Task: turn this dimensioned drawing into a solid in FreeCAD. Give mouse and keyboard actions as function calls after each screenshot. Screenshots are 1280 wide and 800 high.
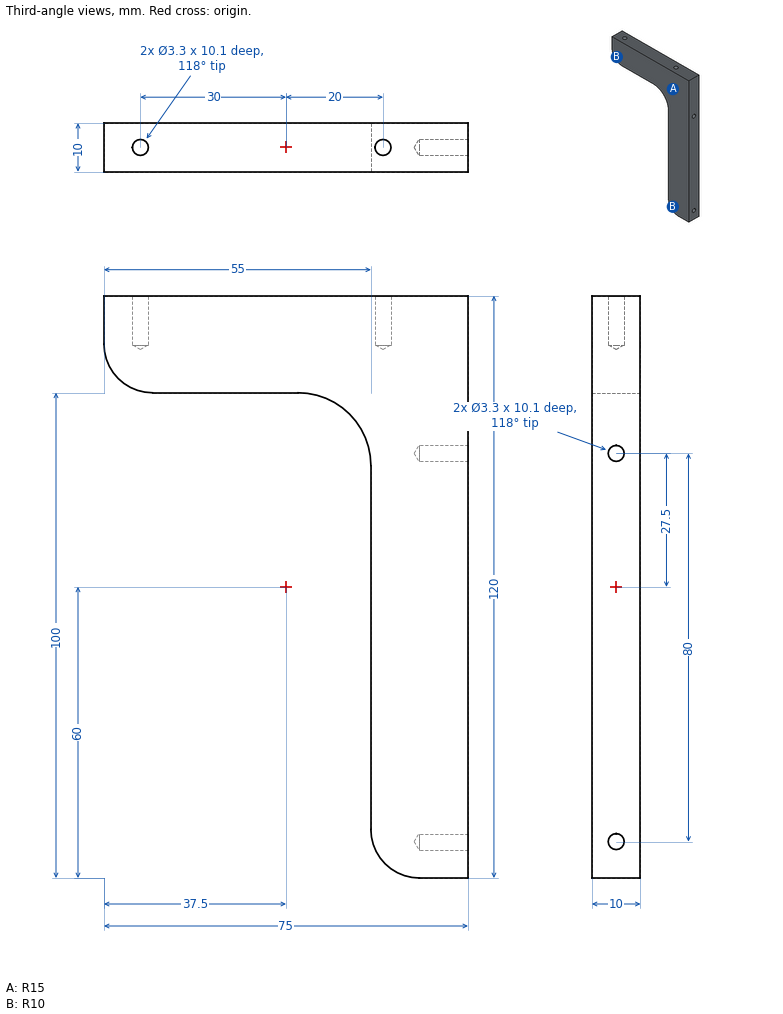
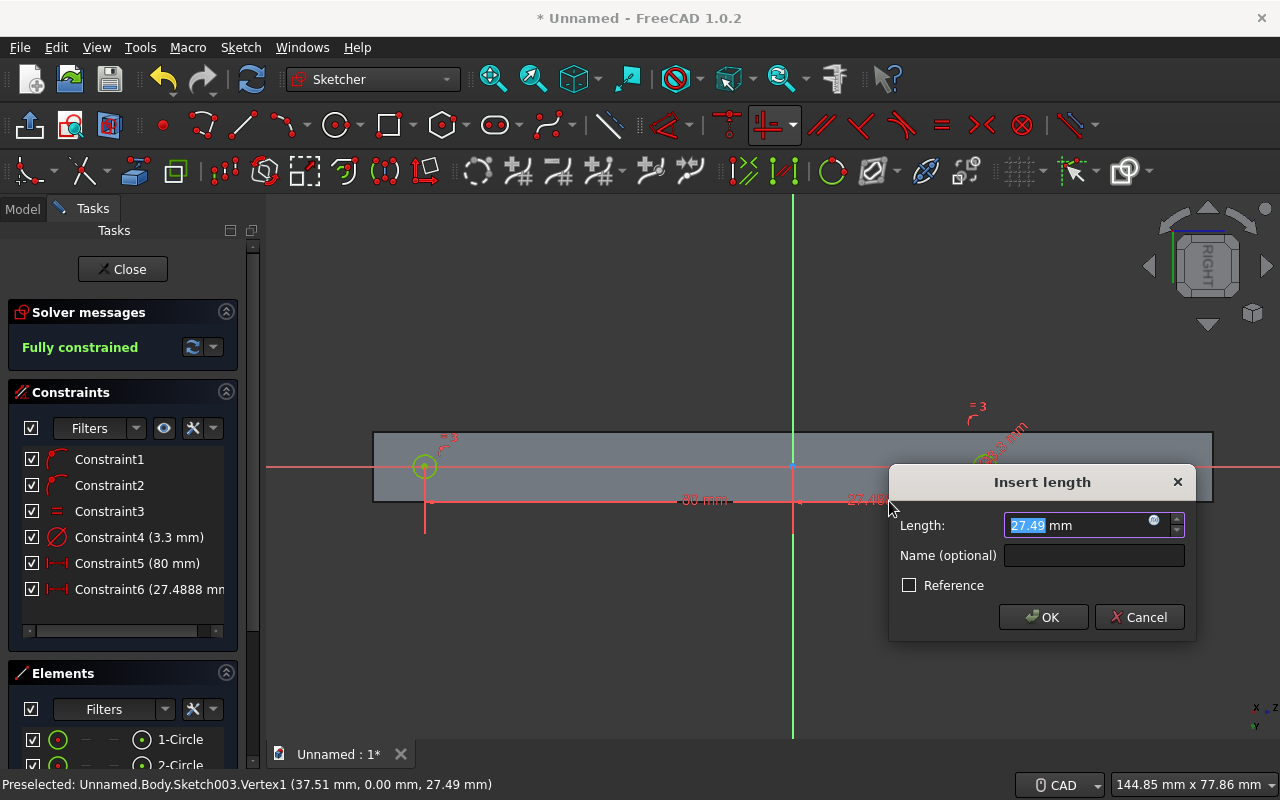
text(27.5)
key(Return)
key(Escape)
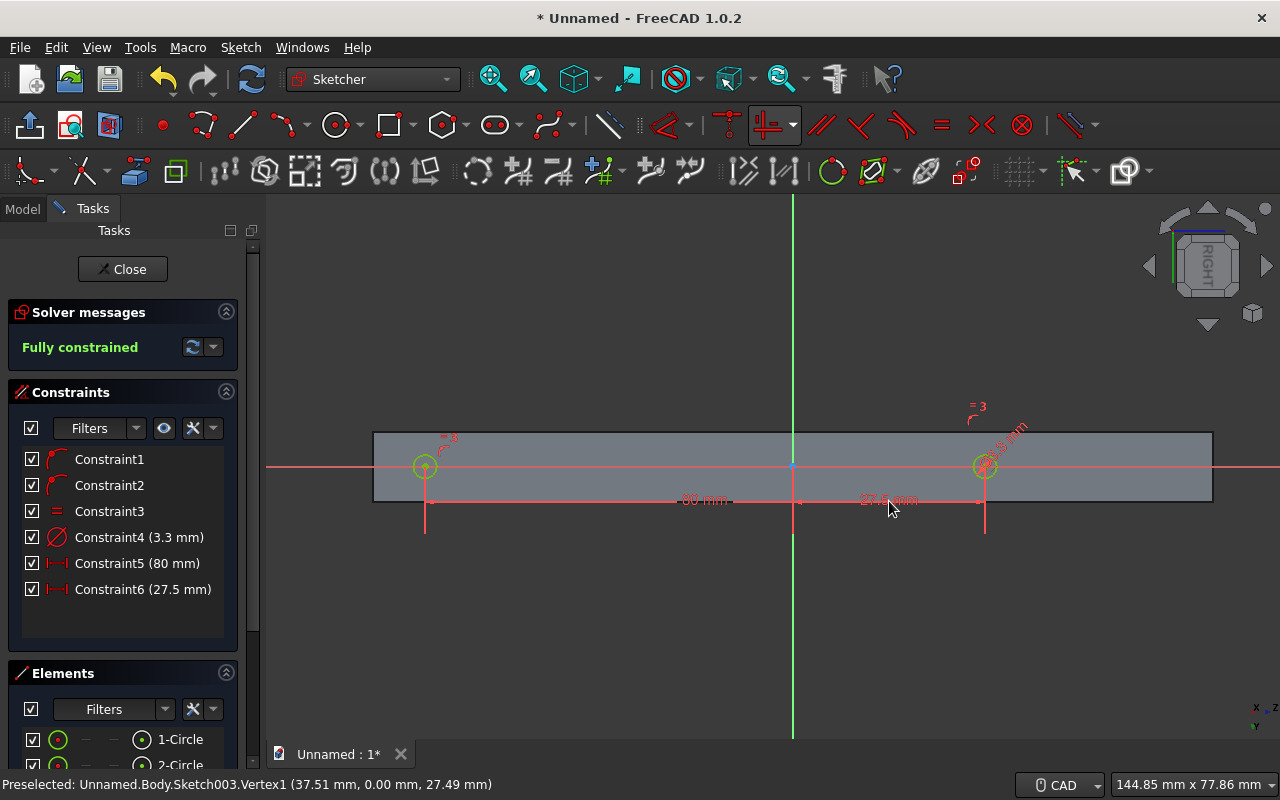
click(123, 269)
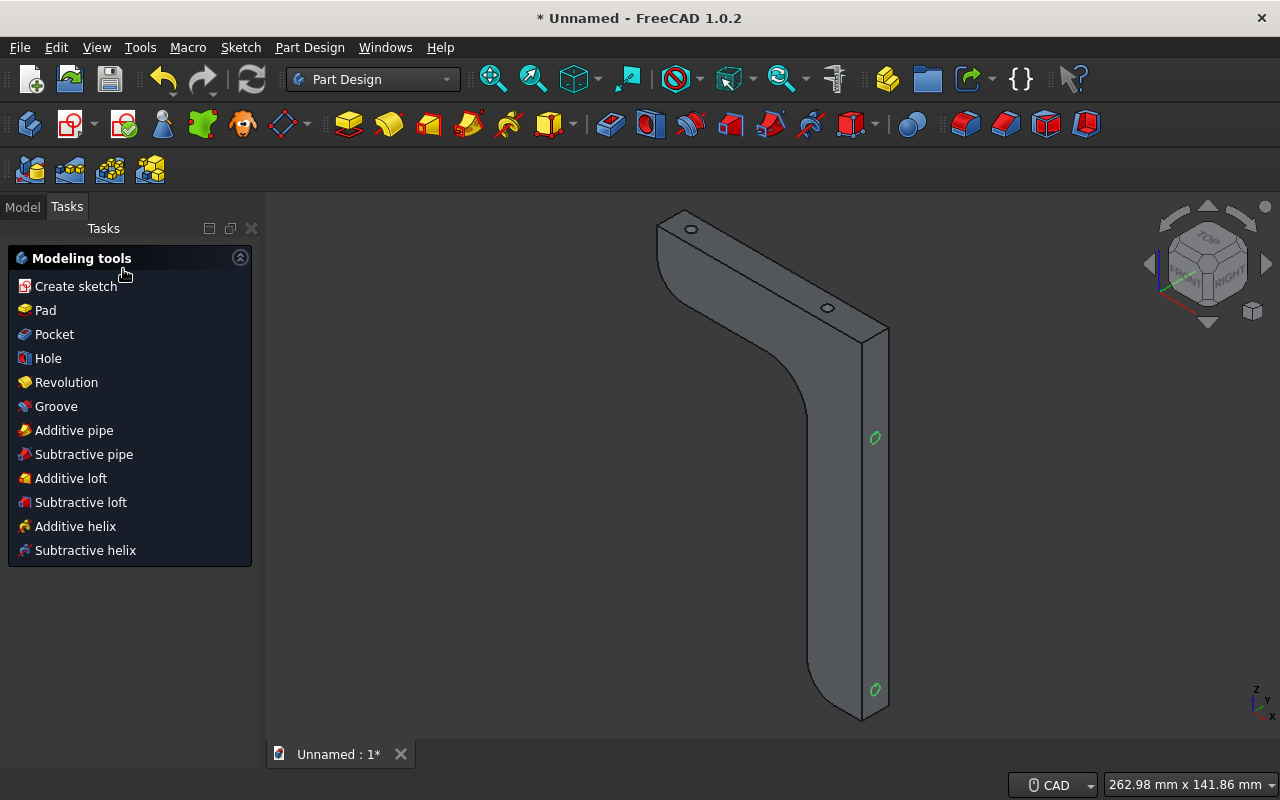
click(652, 124)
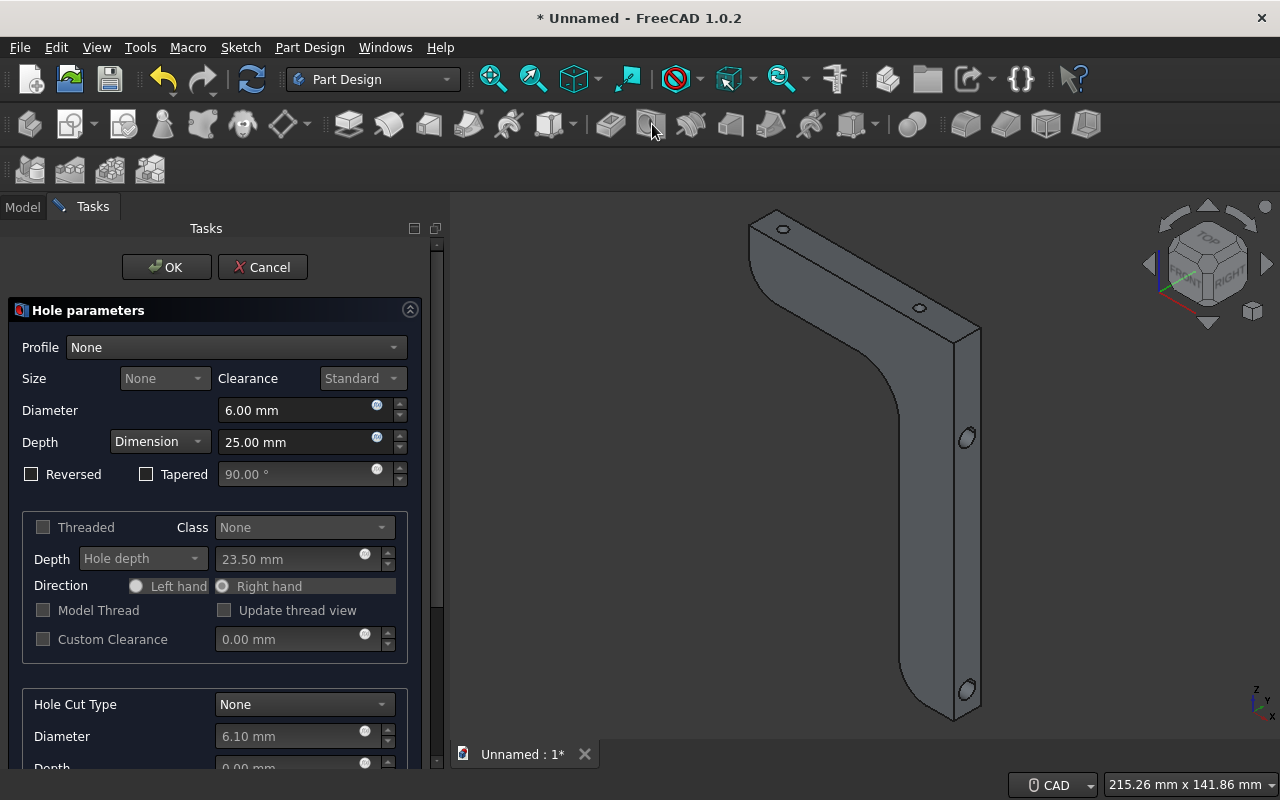
triple_click(305, 410)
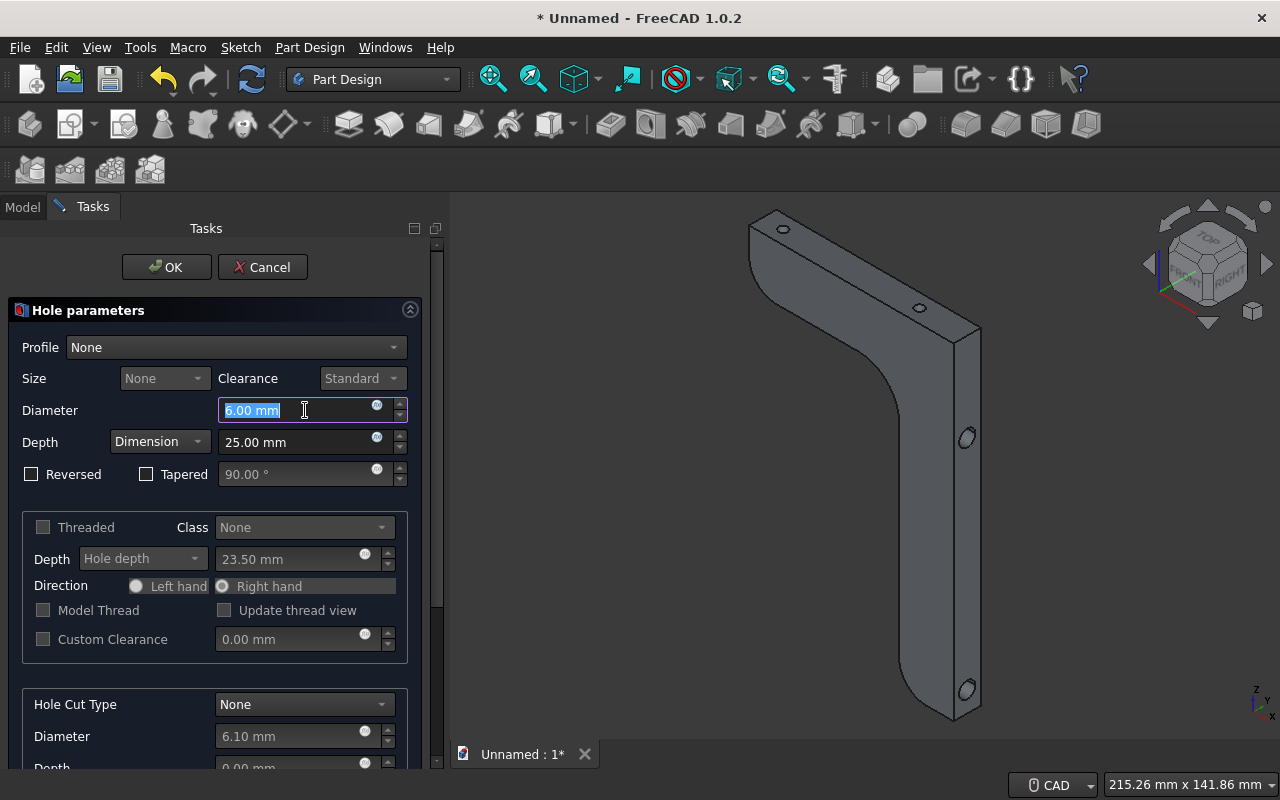
text(3.3)
key(Tab)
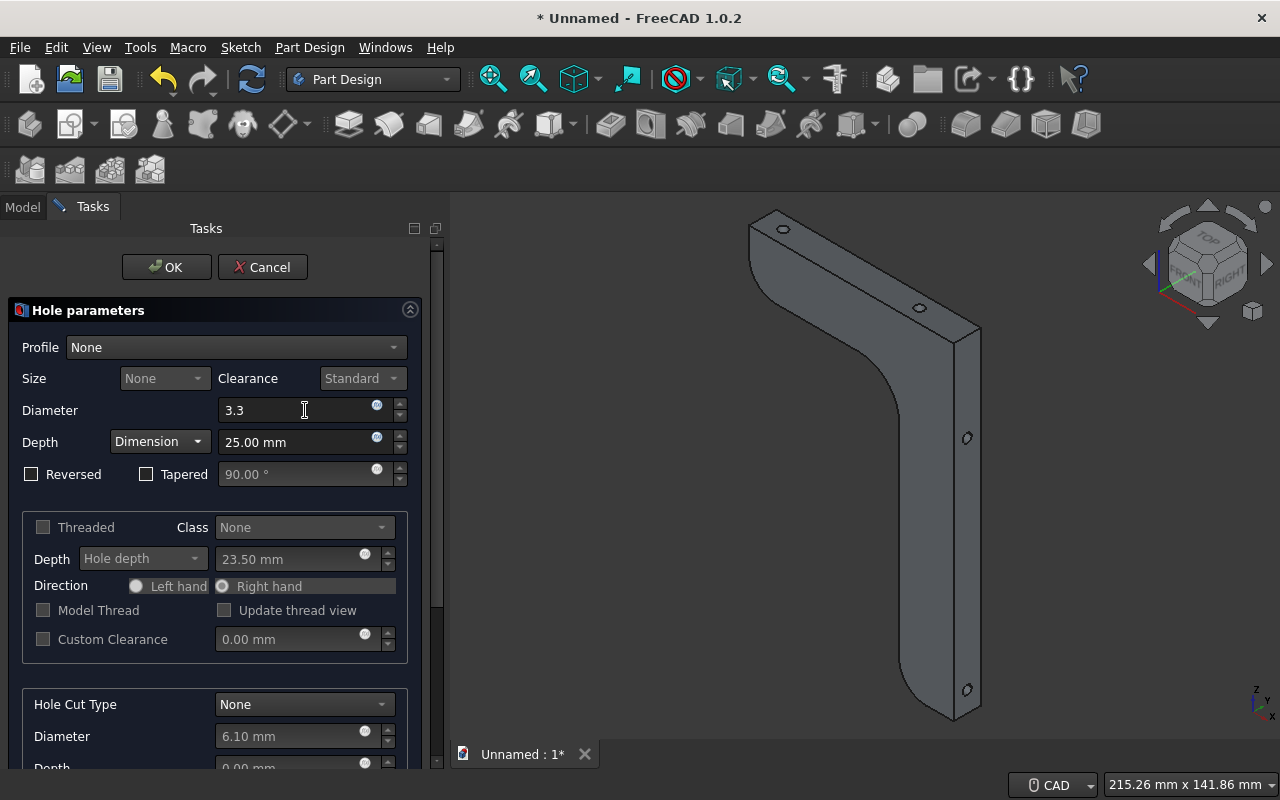
triple_click(305, 442)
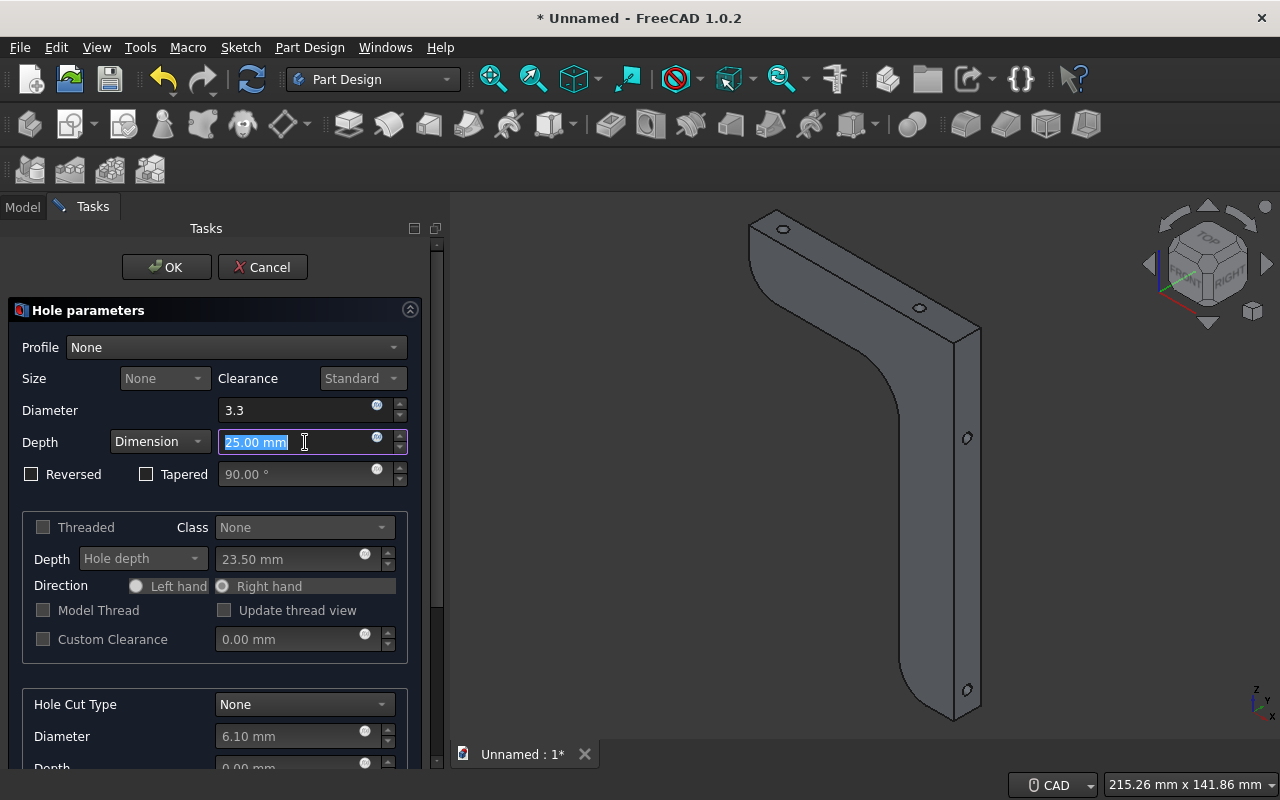
text(10.1)
key(Tab)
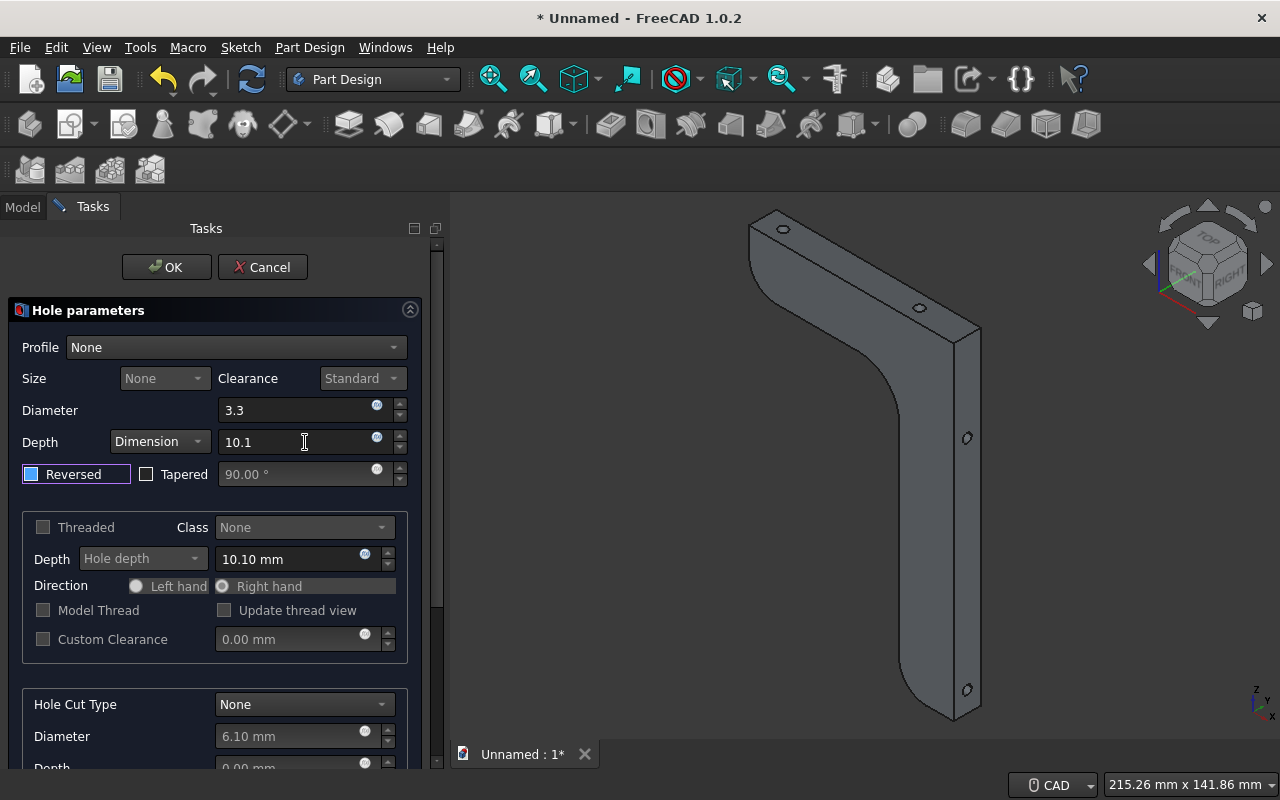
click(167, 267)